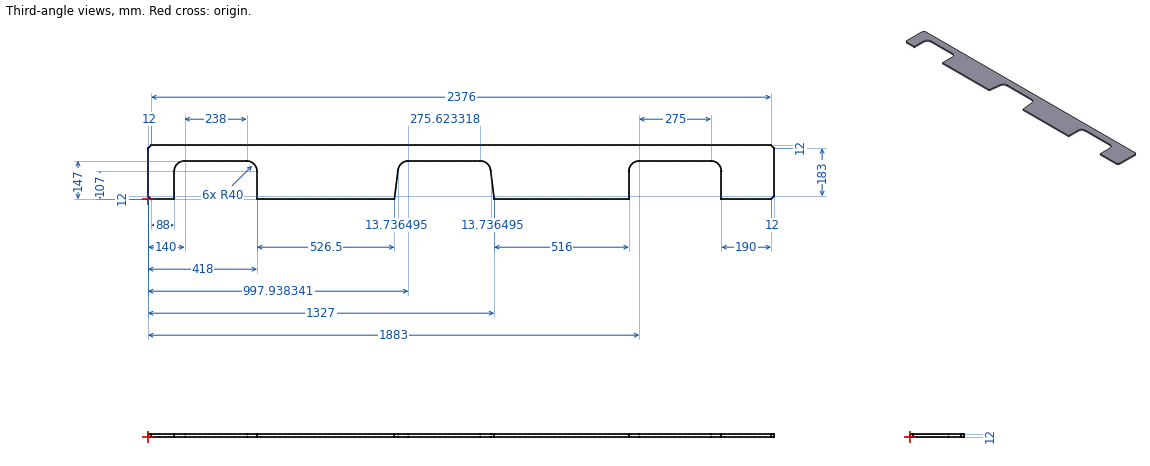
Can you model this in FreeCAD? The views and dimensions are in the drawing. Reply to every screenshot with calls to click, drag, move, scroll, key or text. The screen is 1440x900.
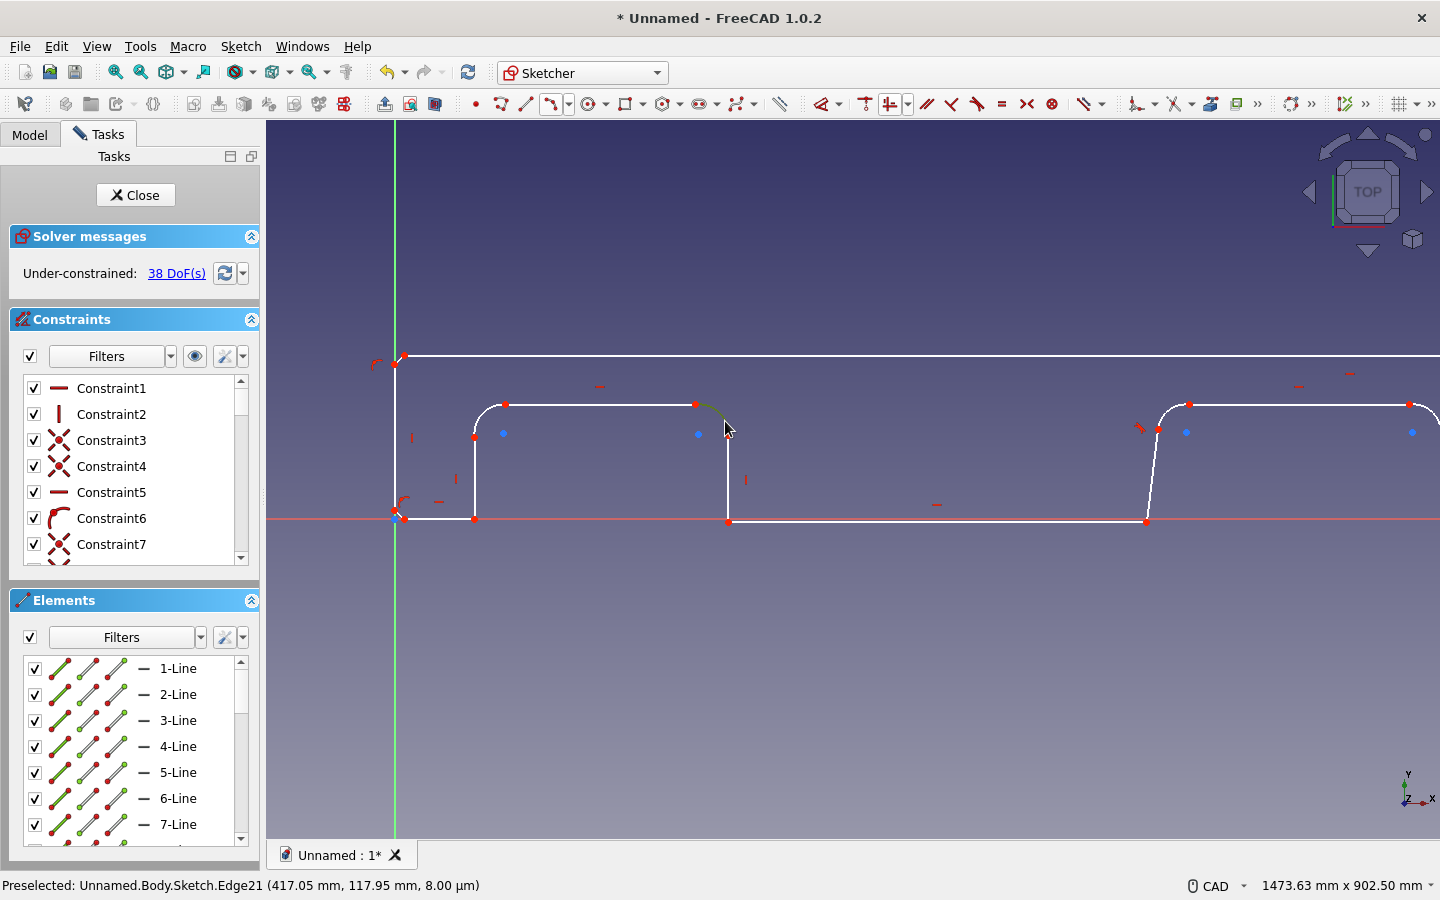
click(1176, 406)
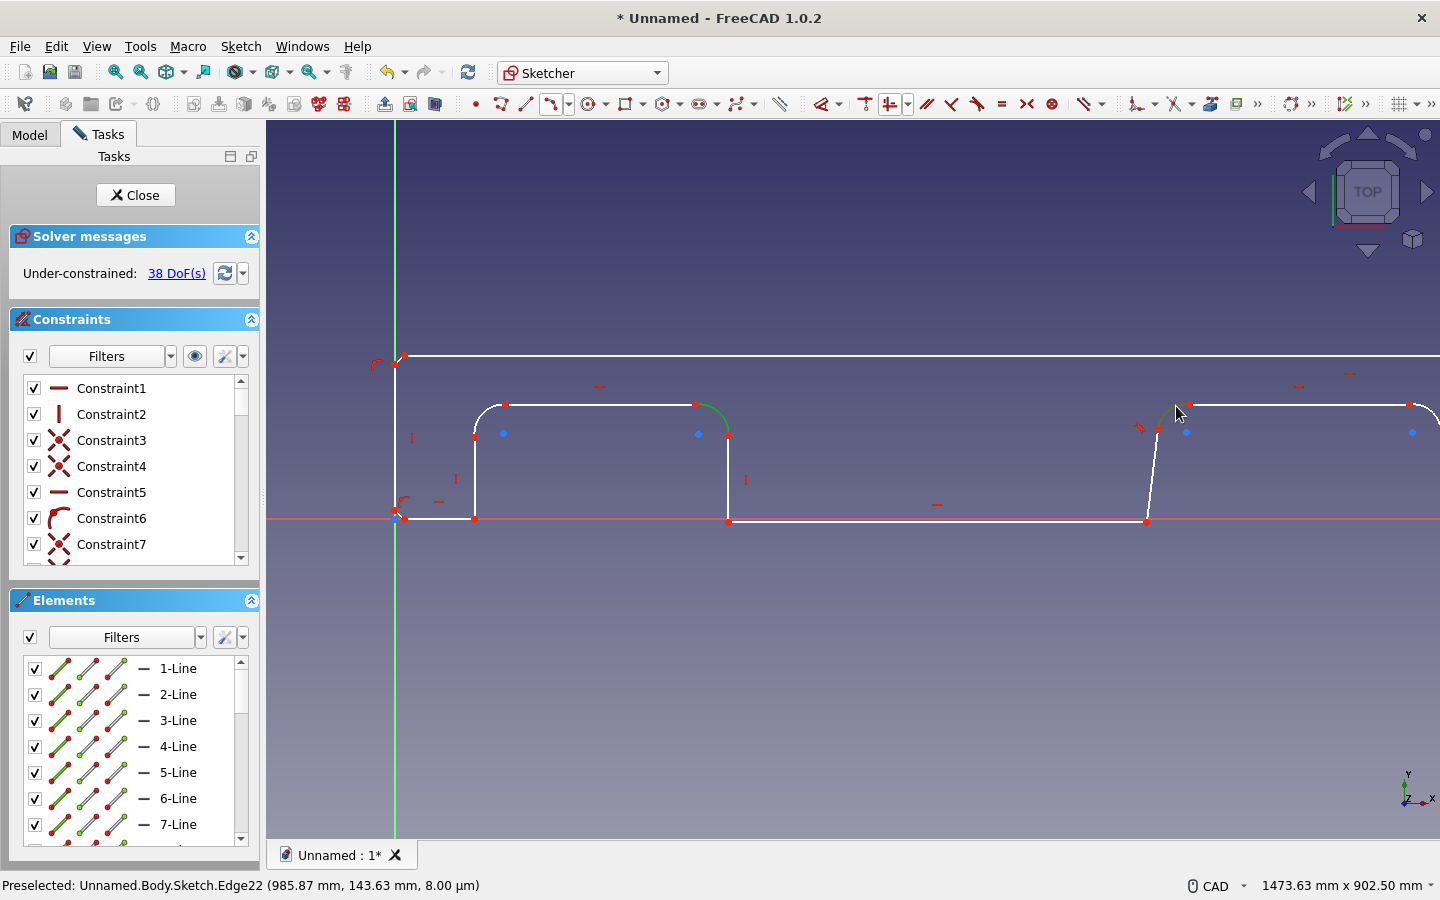
scroll(455, 504, down, 5)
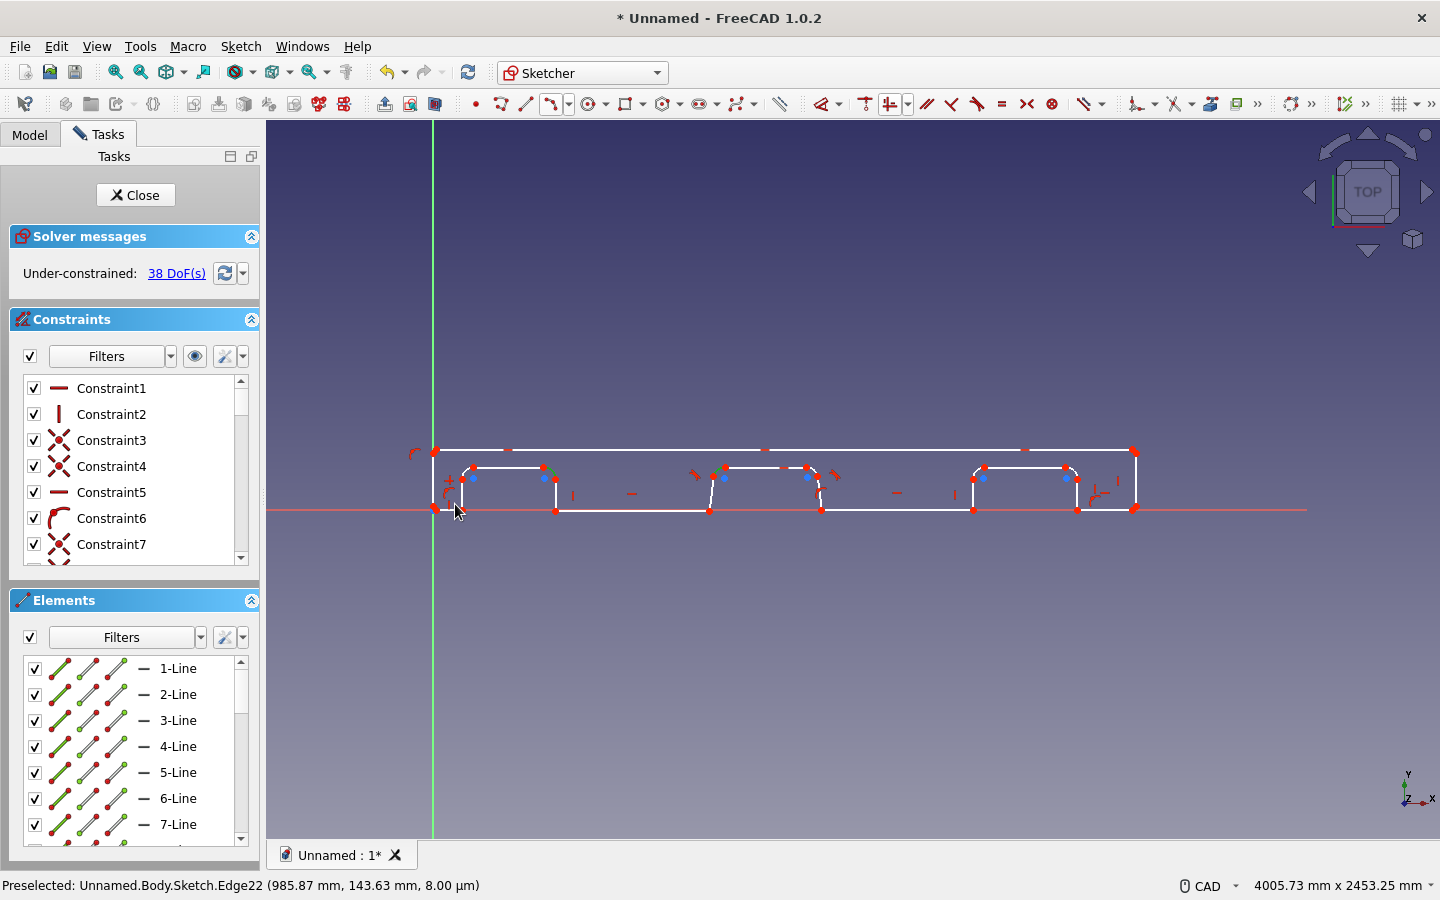
scroll(816, 472, up, 6)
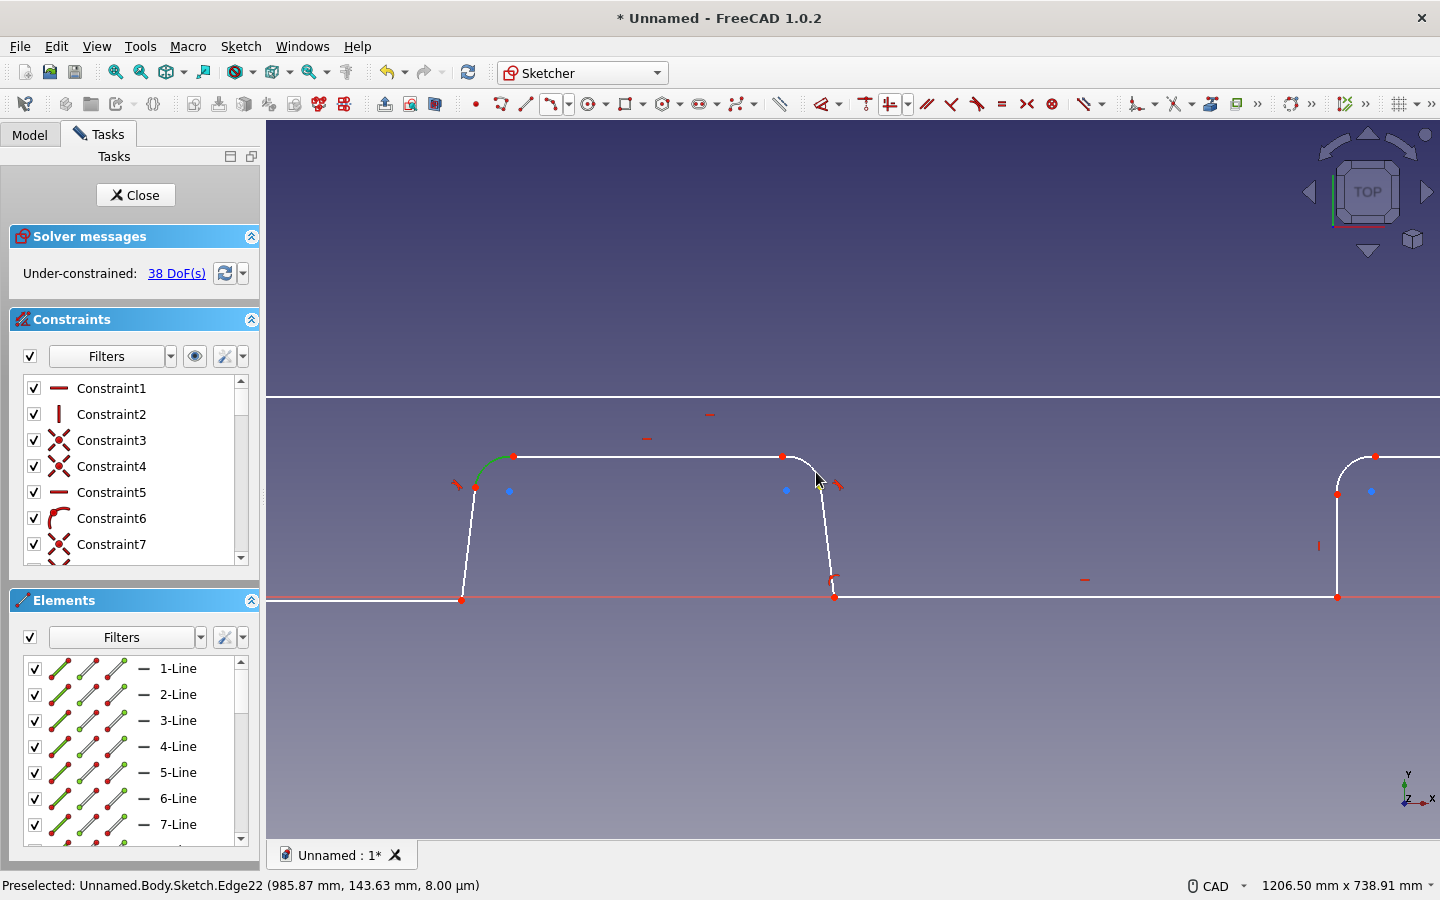
click(815, 472)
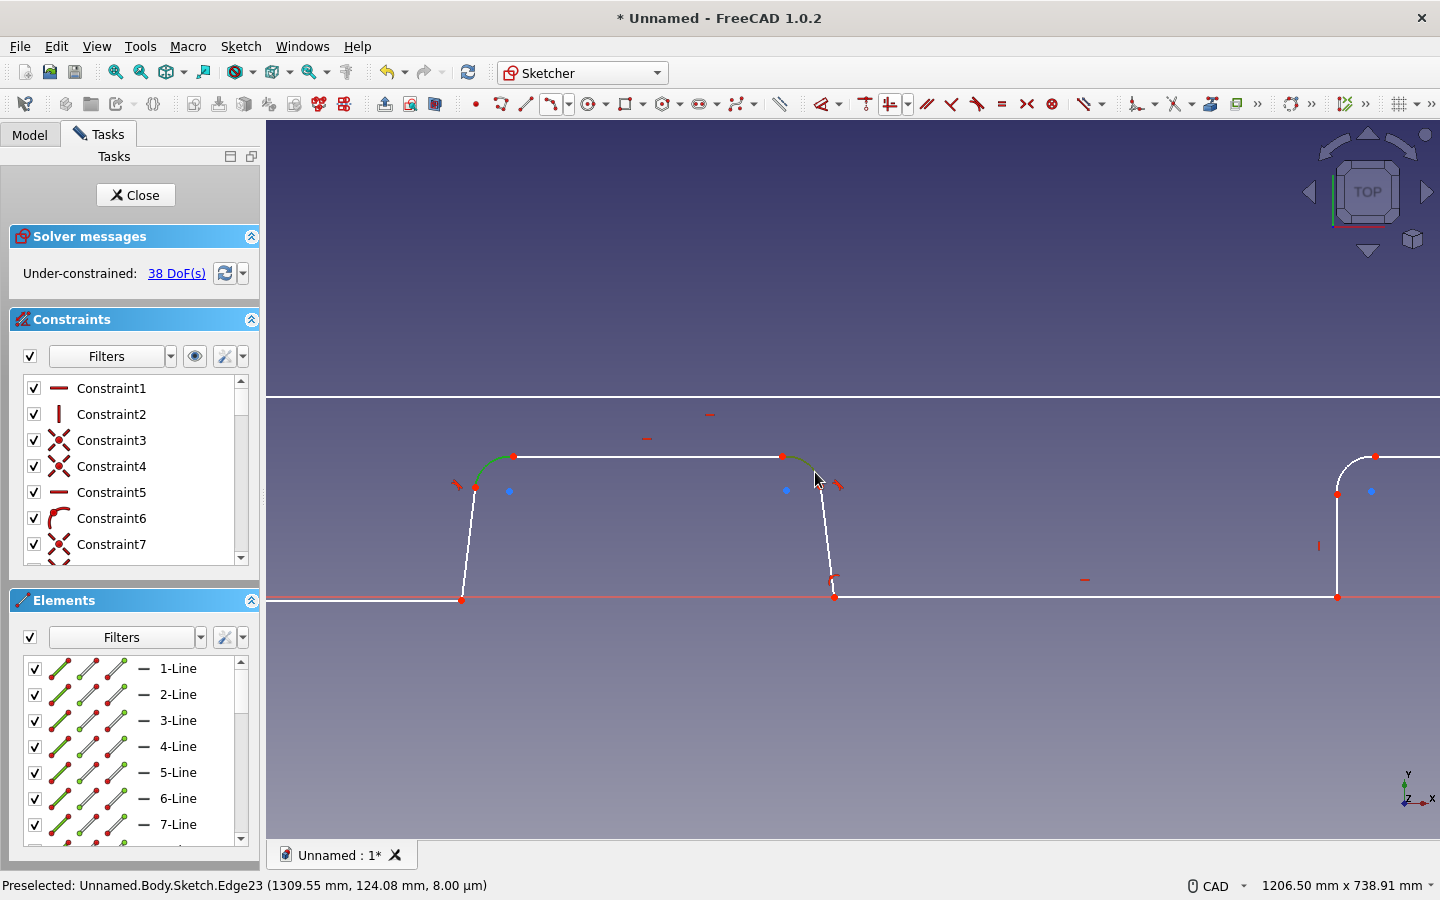
scroll(816, 472, down, 6)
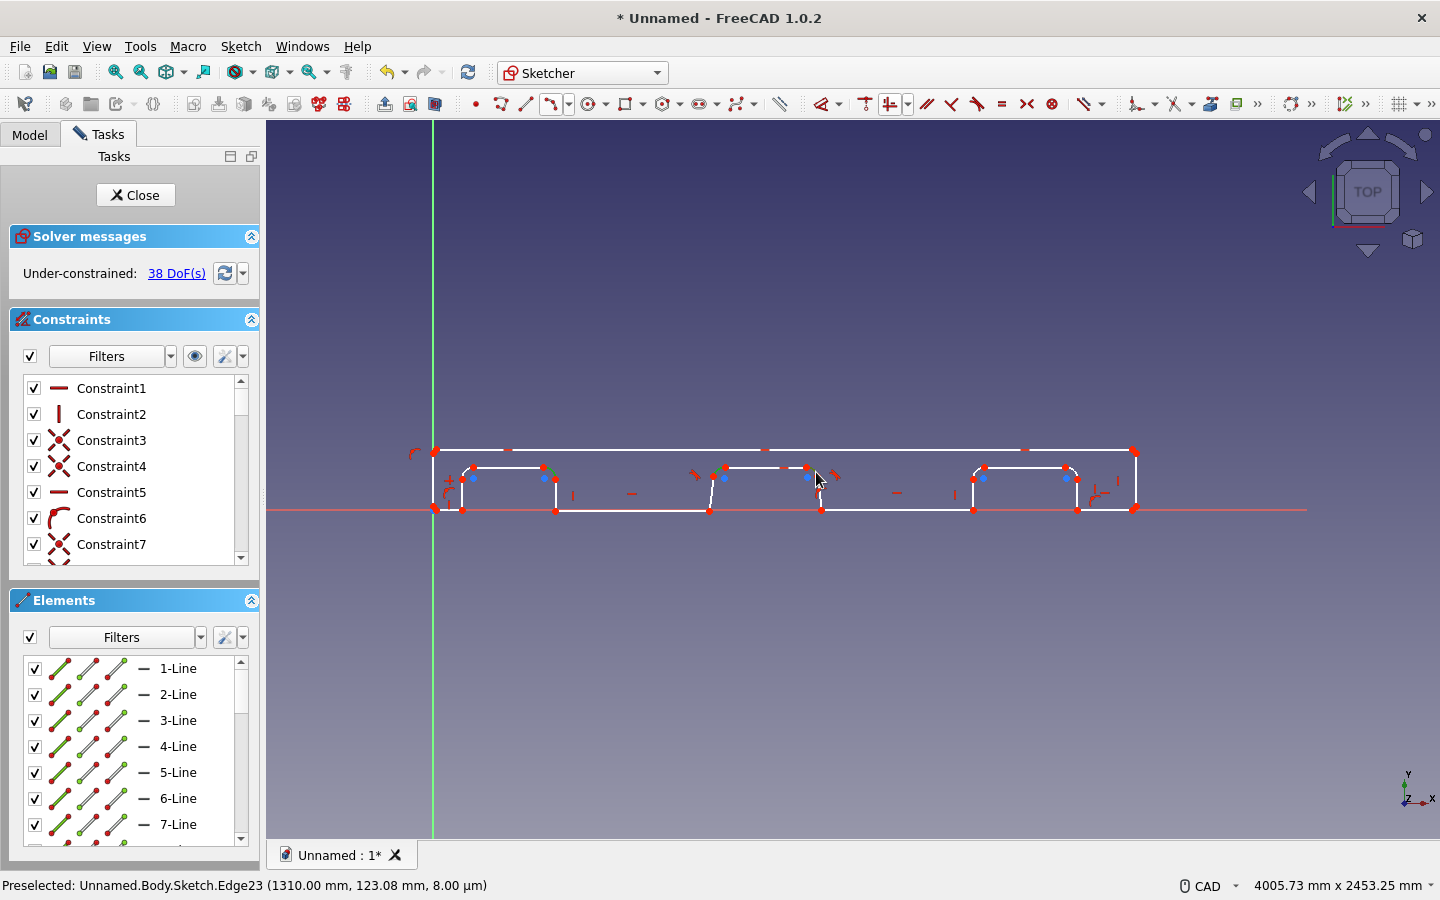
scroll(979, 469, up, 5)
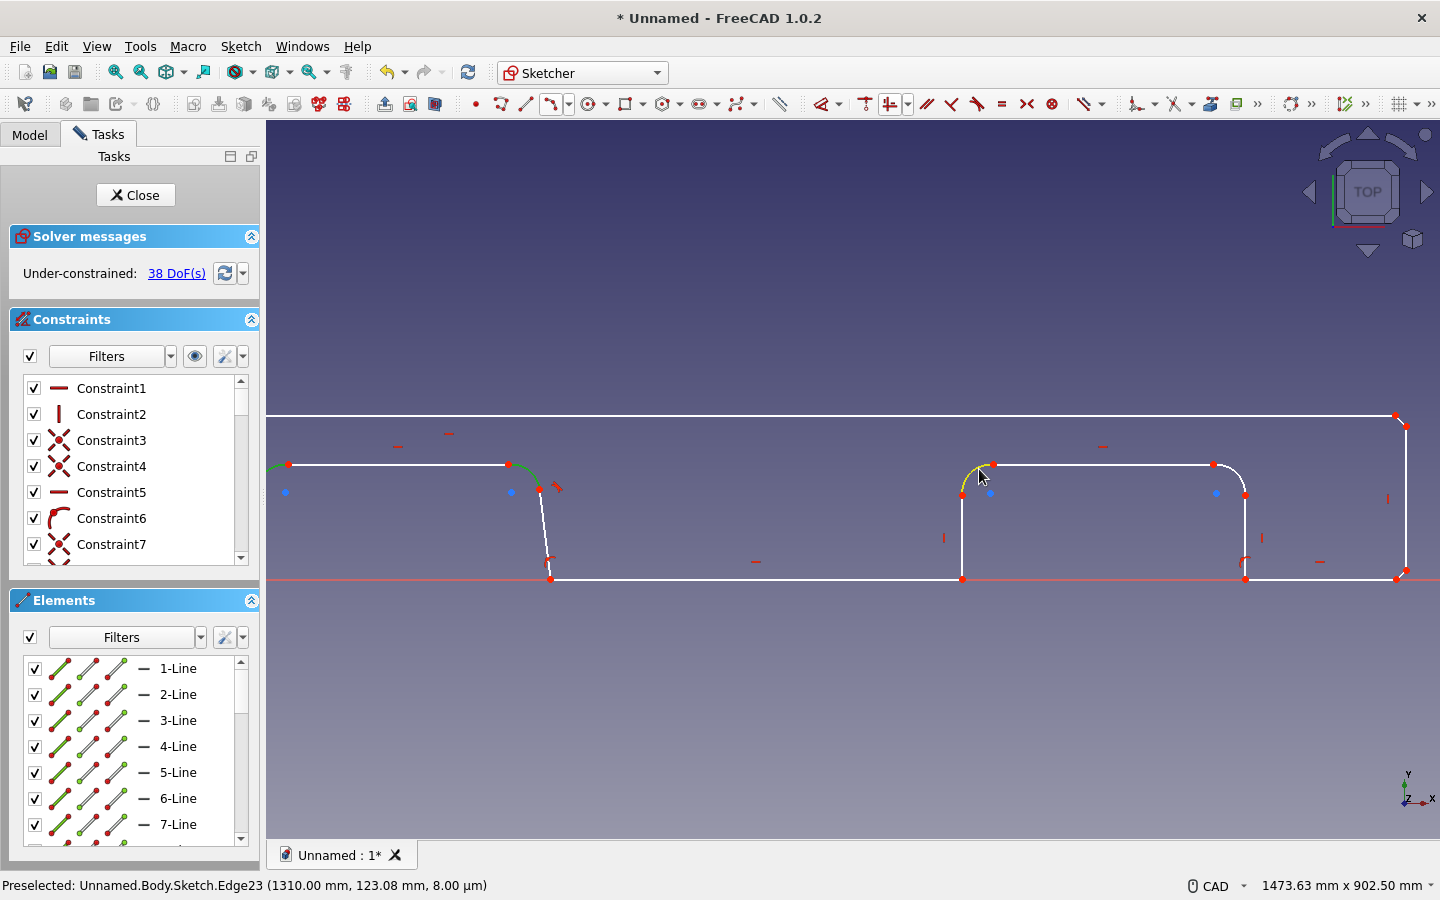
click(979, 467)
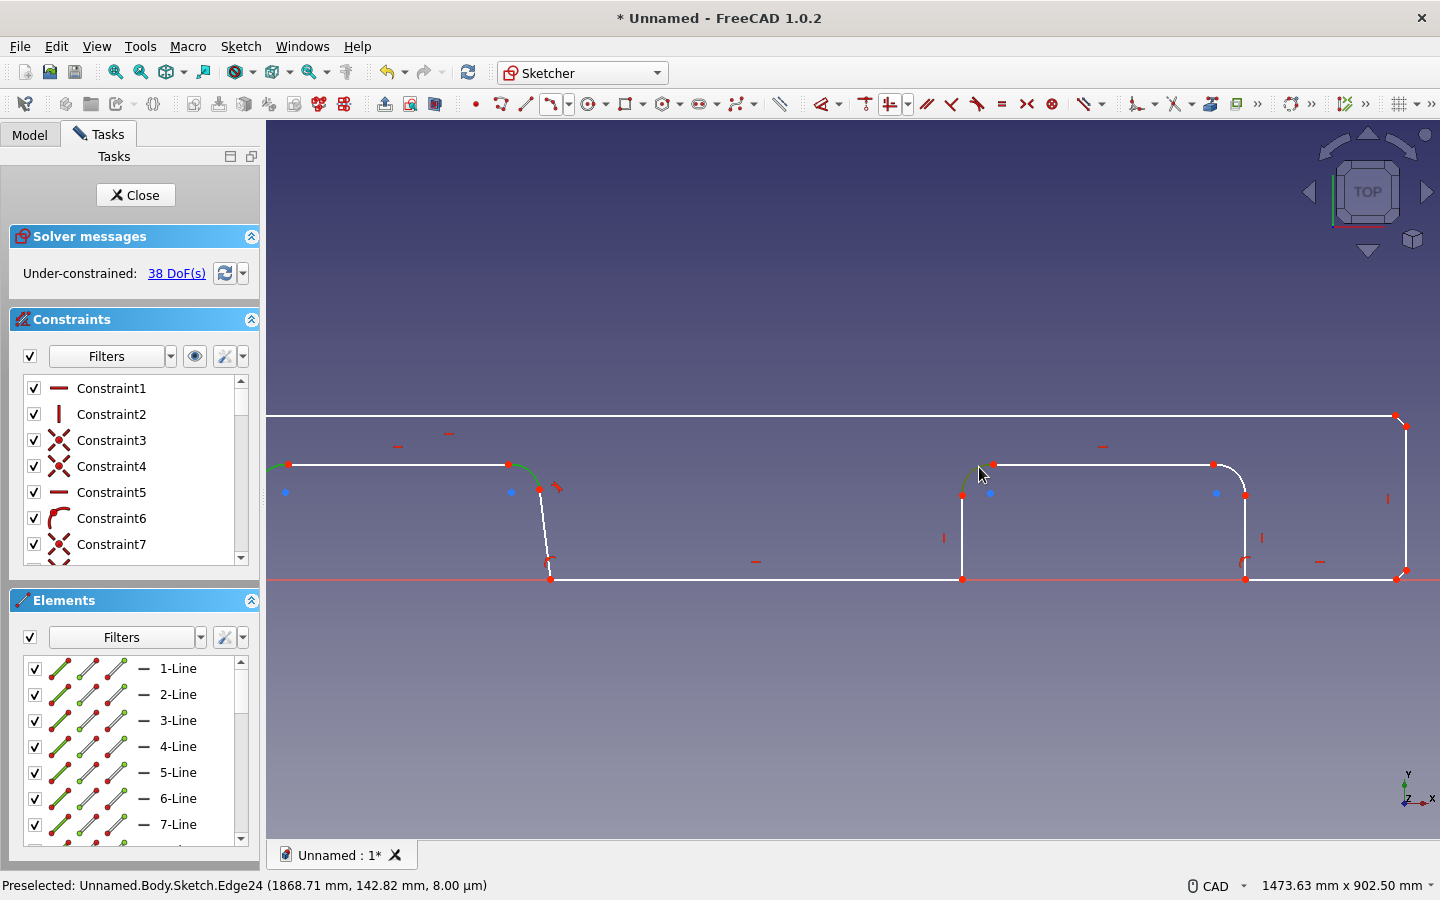
click(1242, 481)